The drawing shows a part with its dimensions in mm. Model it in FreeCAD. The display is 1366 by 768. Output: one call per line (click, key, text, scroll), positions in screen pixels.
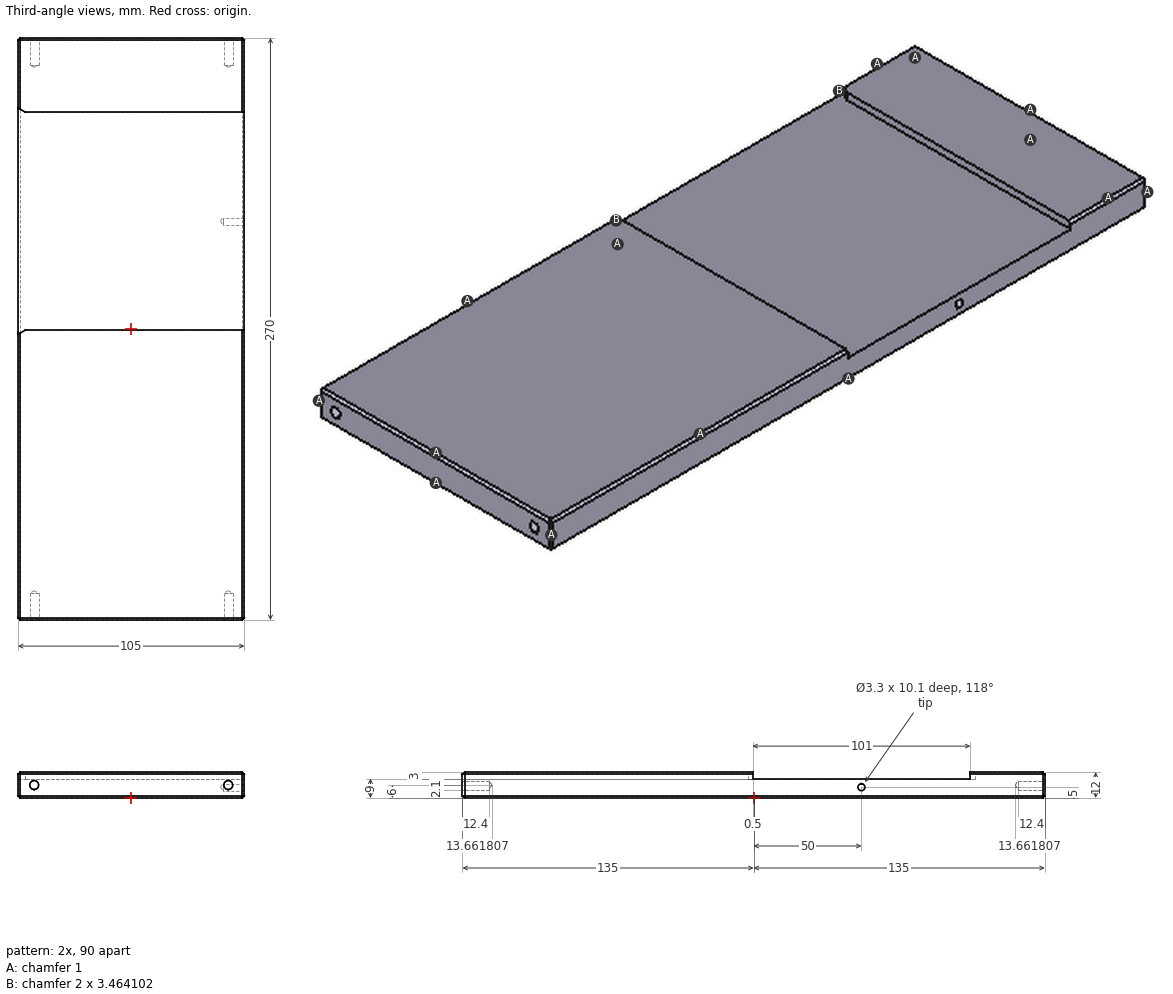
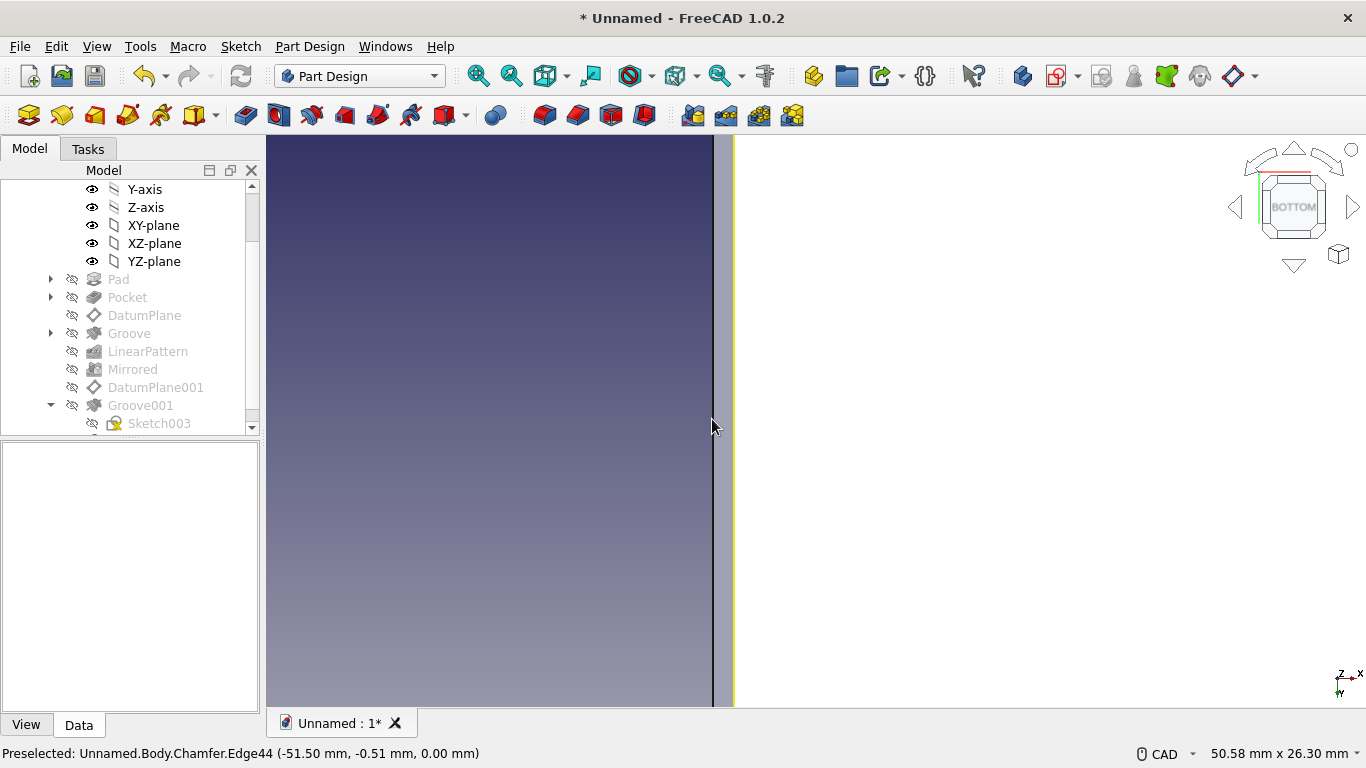
click(479, 76)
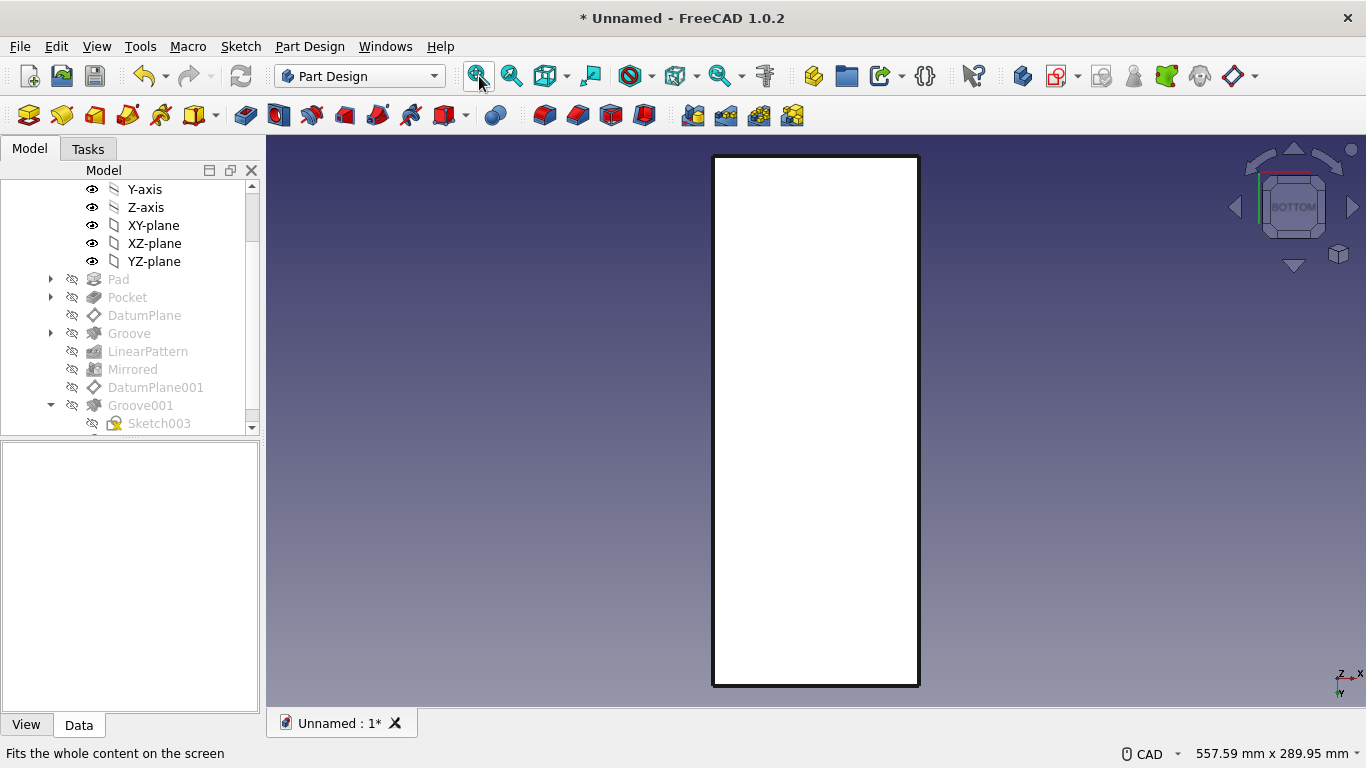
key(4)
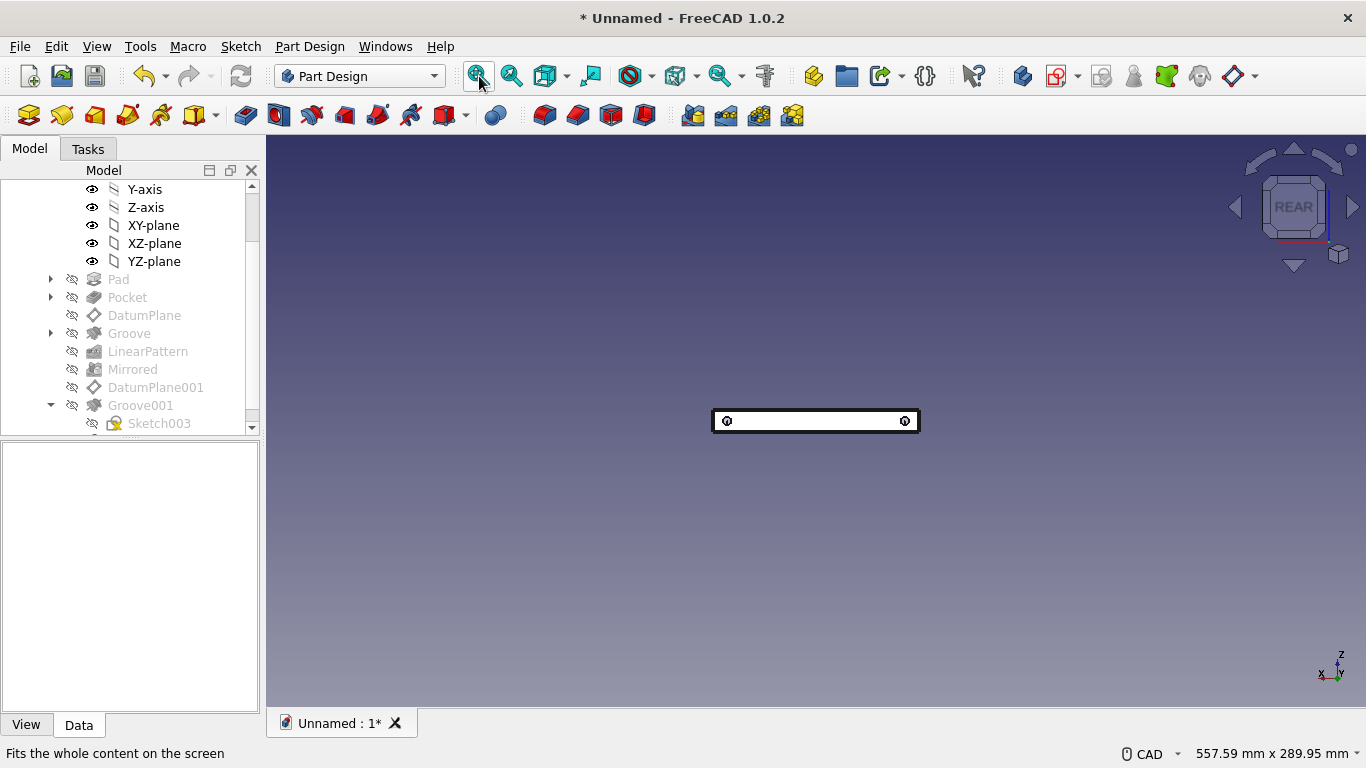
click(479, 76)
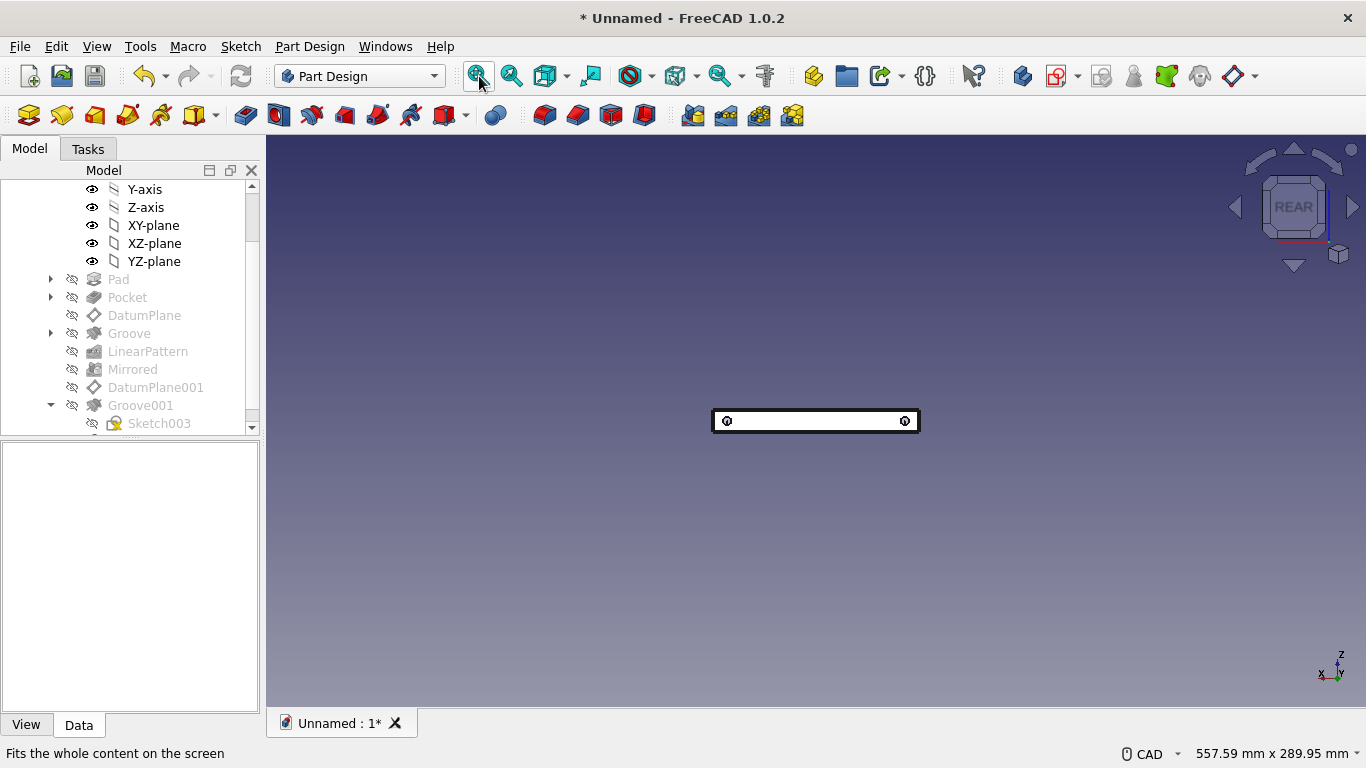
scroll(920, 412, up, 12)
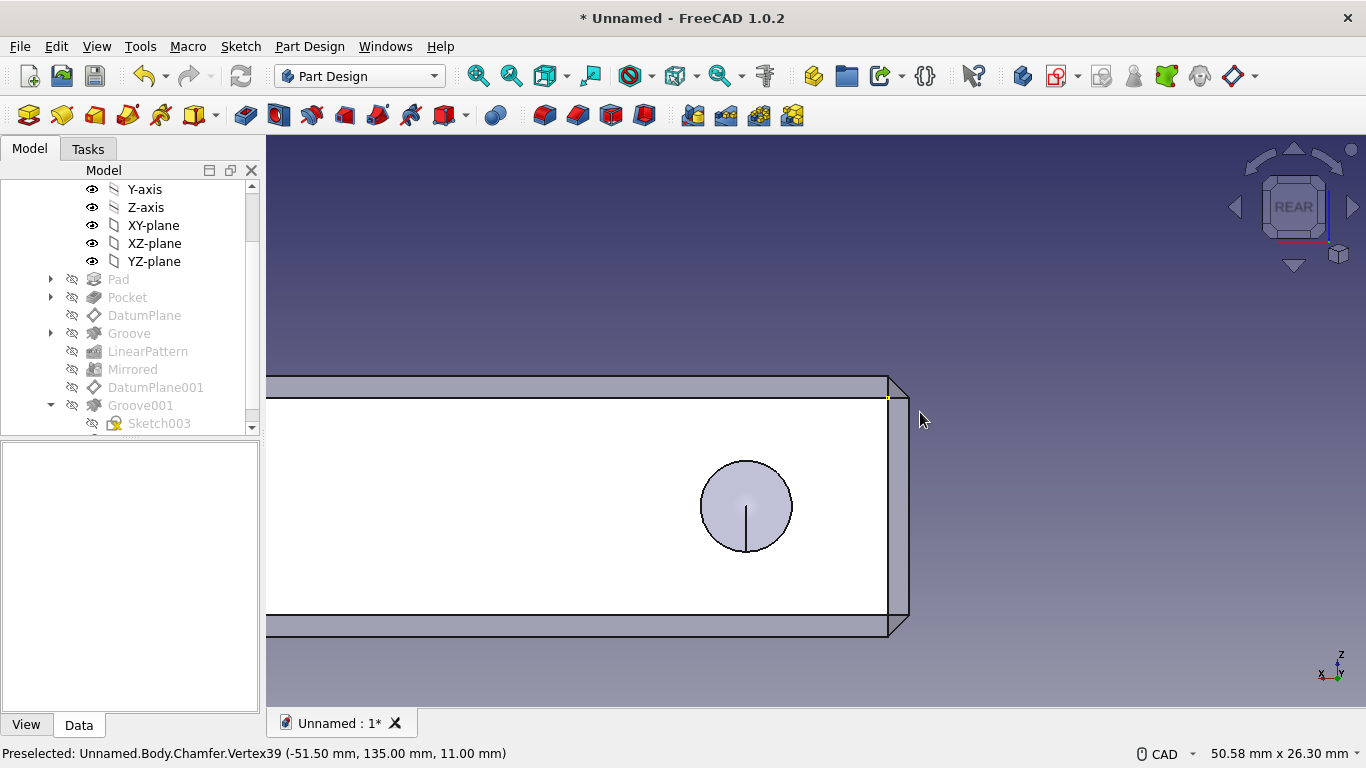
click(479, 76)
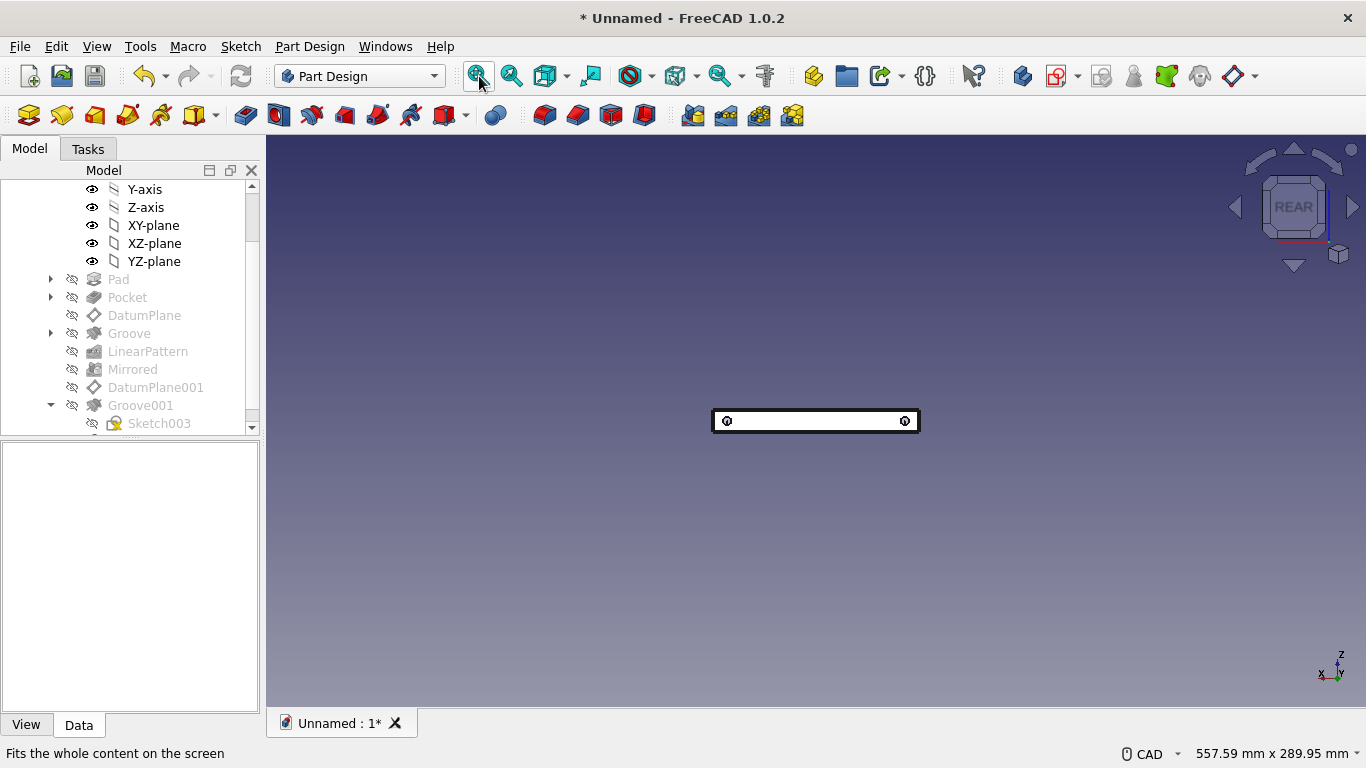
key(6)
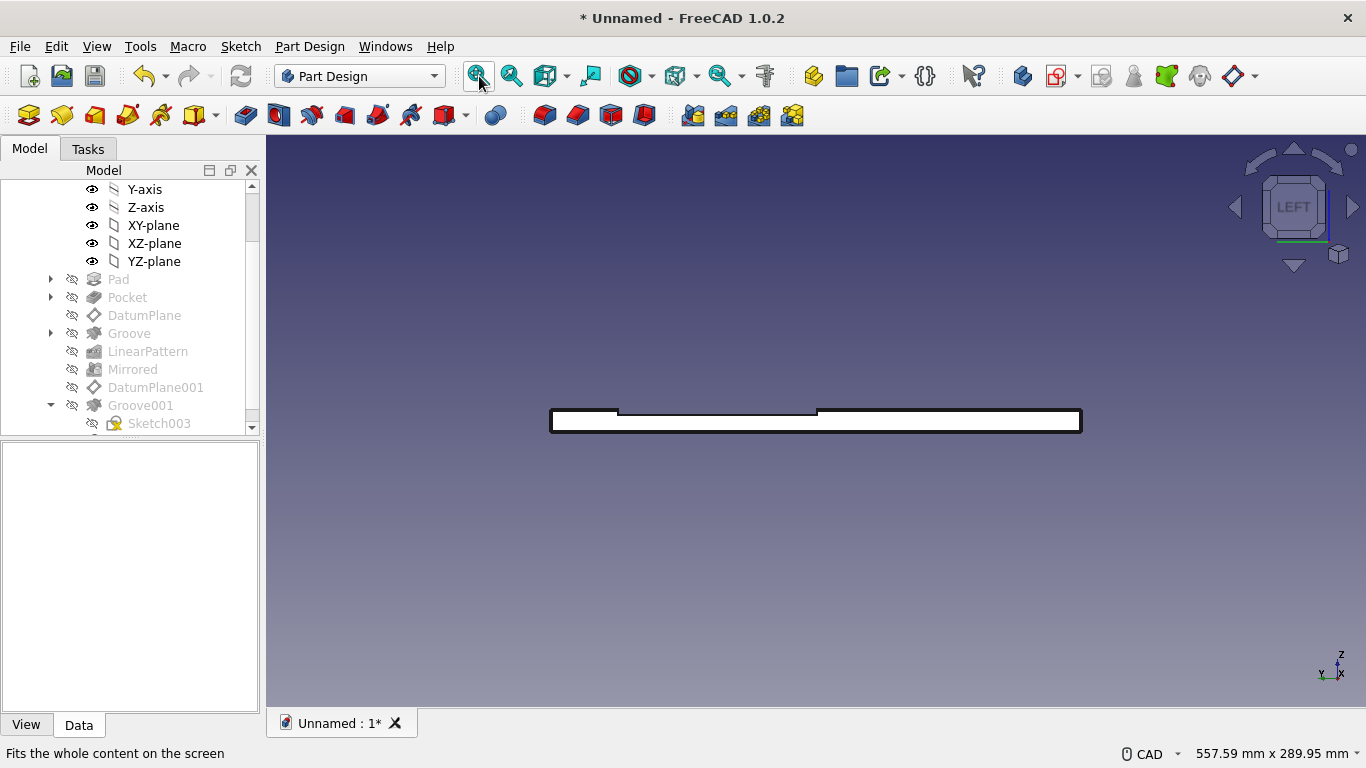
scroll(817, 412, up, 12)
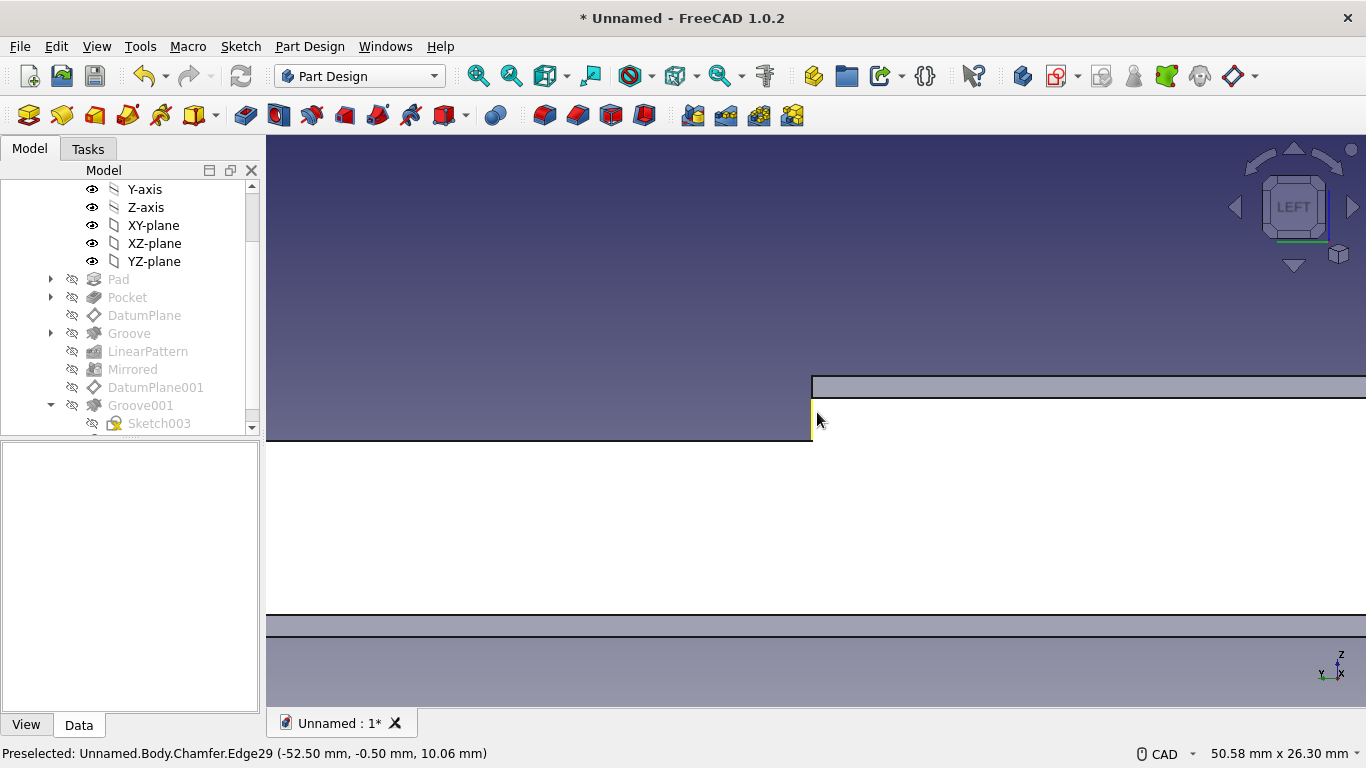
click(812, 418)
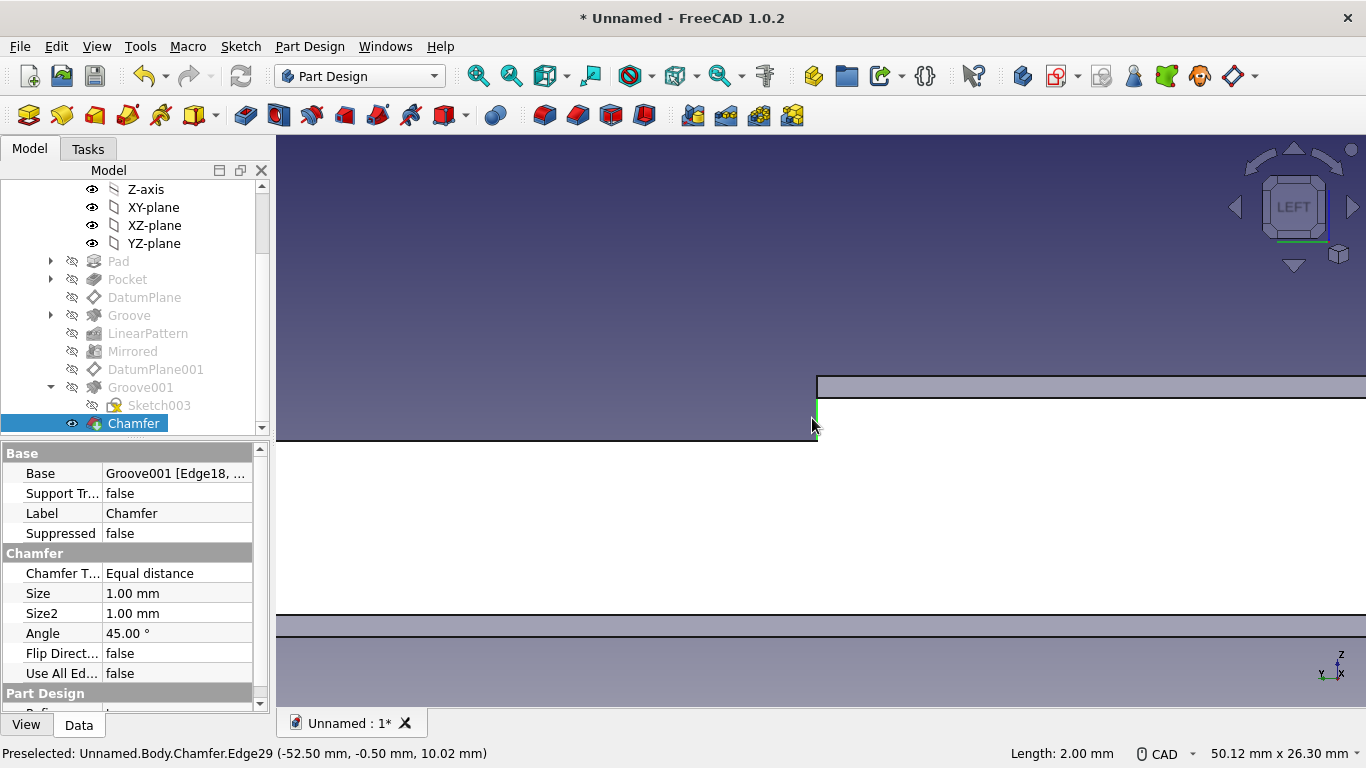
click(479, 76)